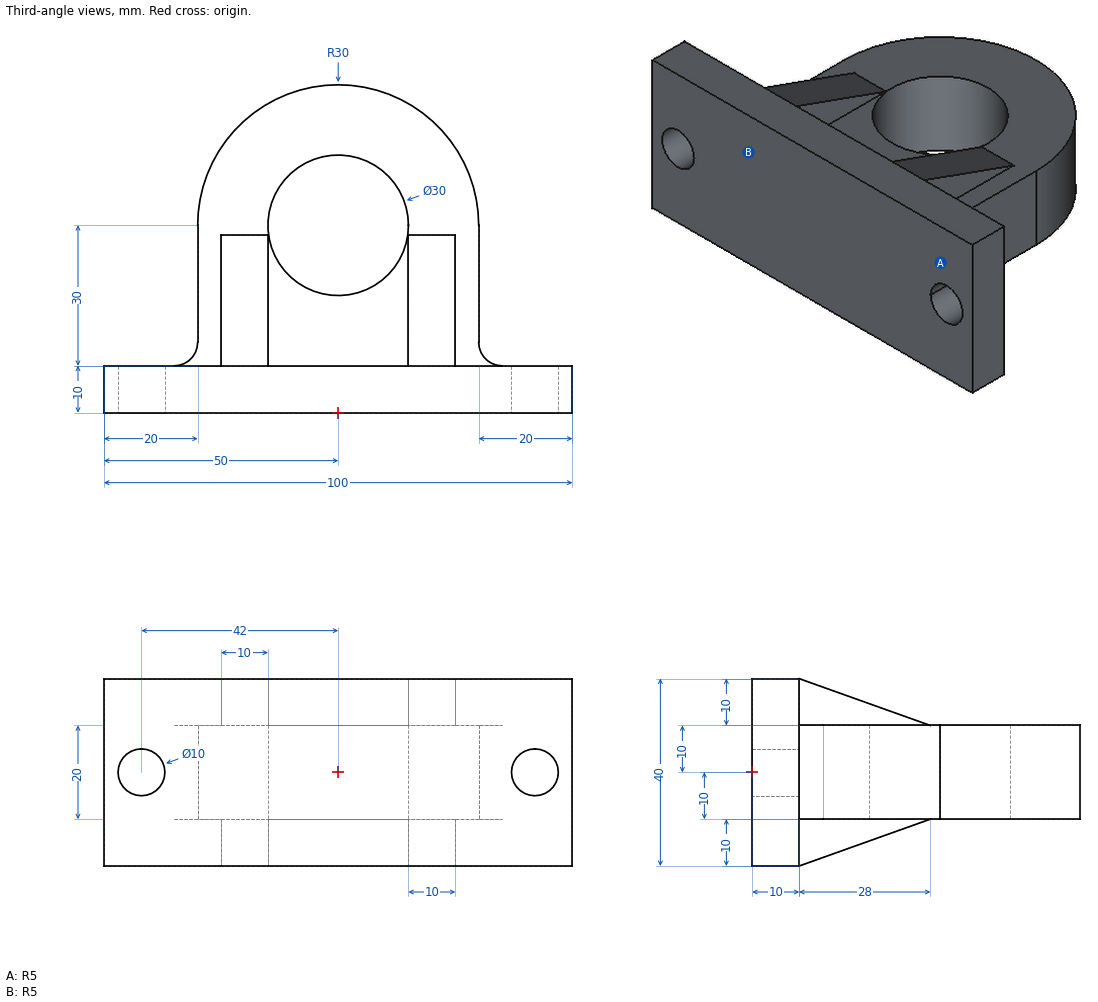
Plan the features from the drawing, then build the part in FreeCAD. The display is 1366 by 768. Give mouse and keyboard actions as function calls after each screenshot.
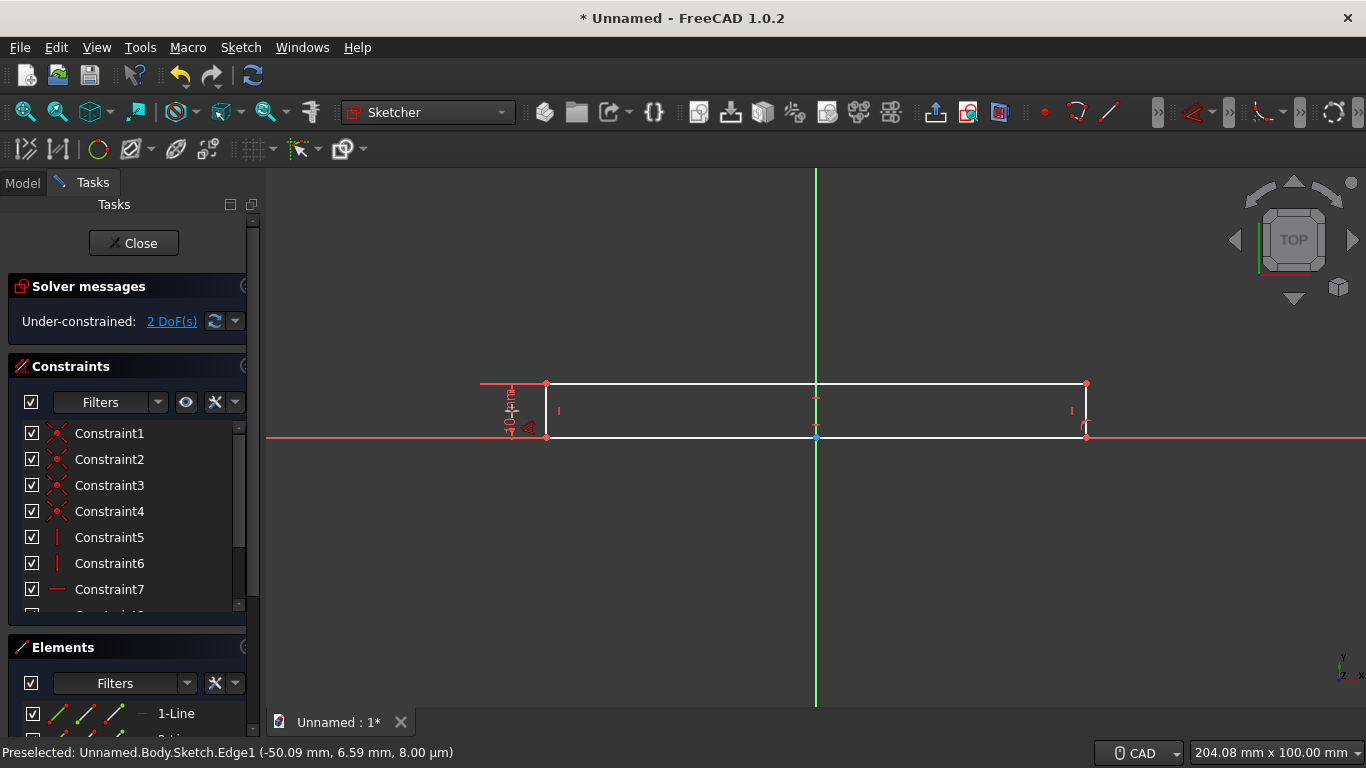
click(708, 438)
click(692, 472)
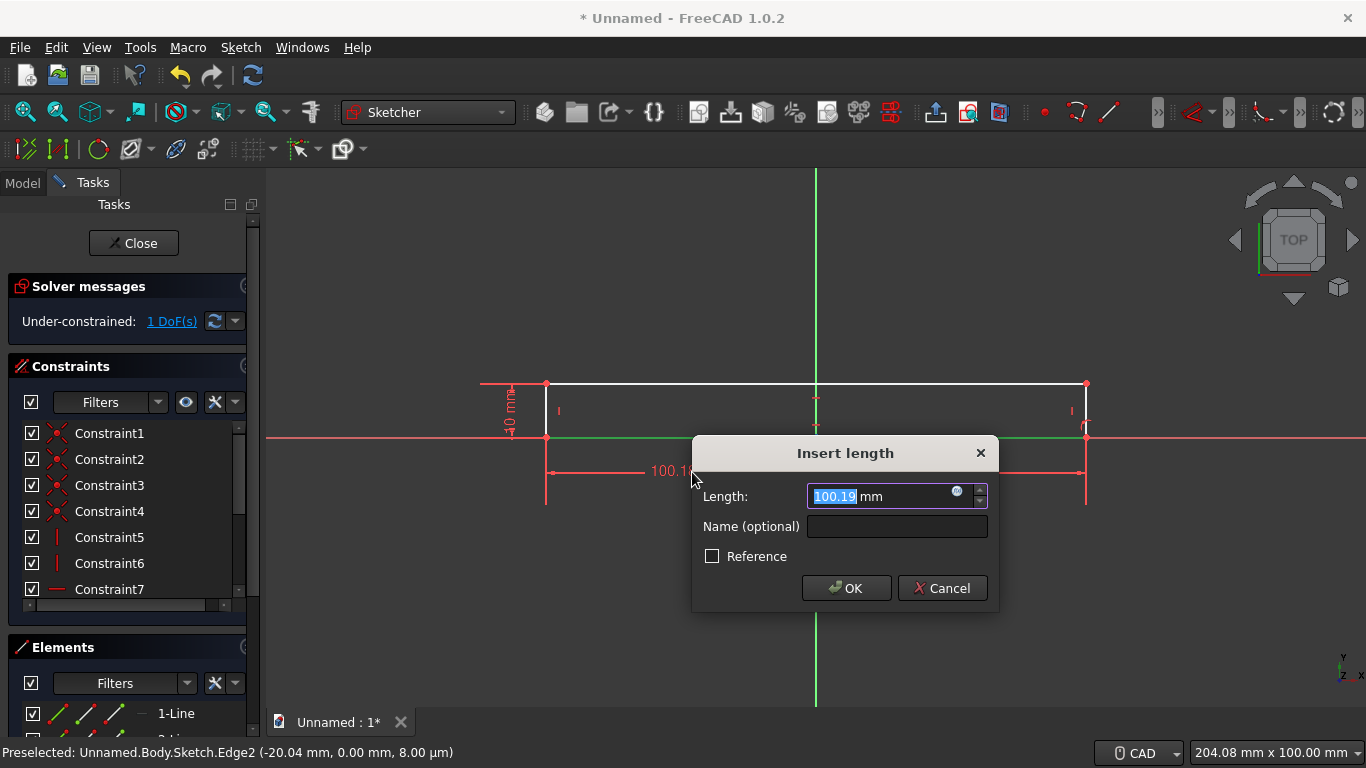
text(100)
key(Return)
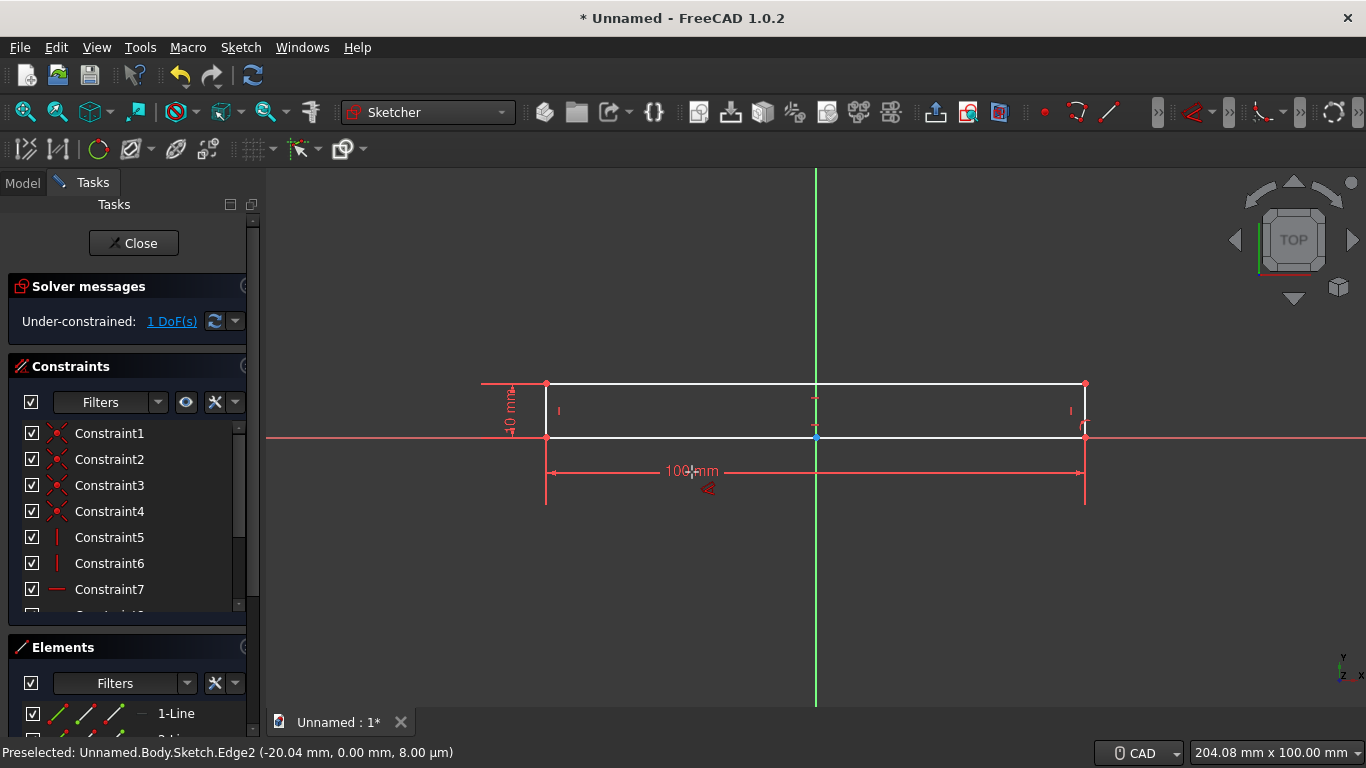
click(546, 384)
click(619, 472)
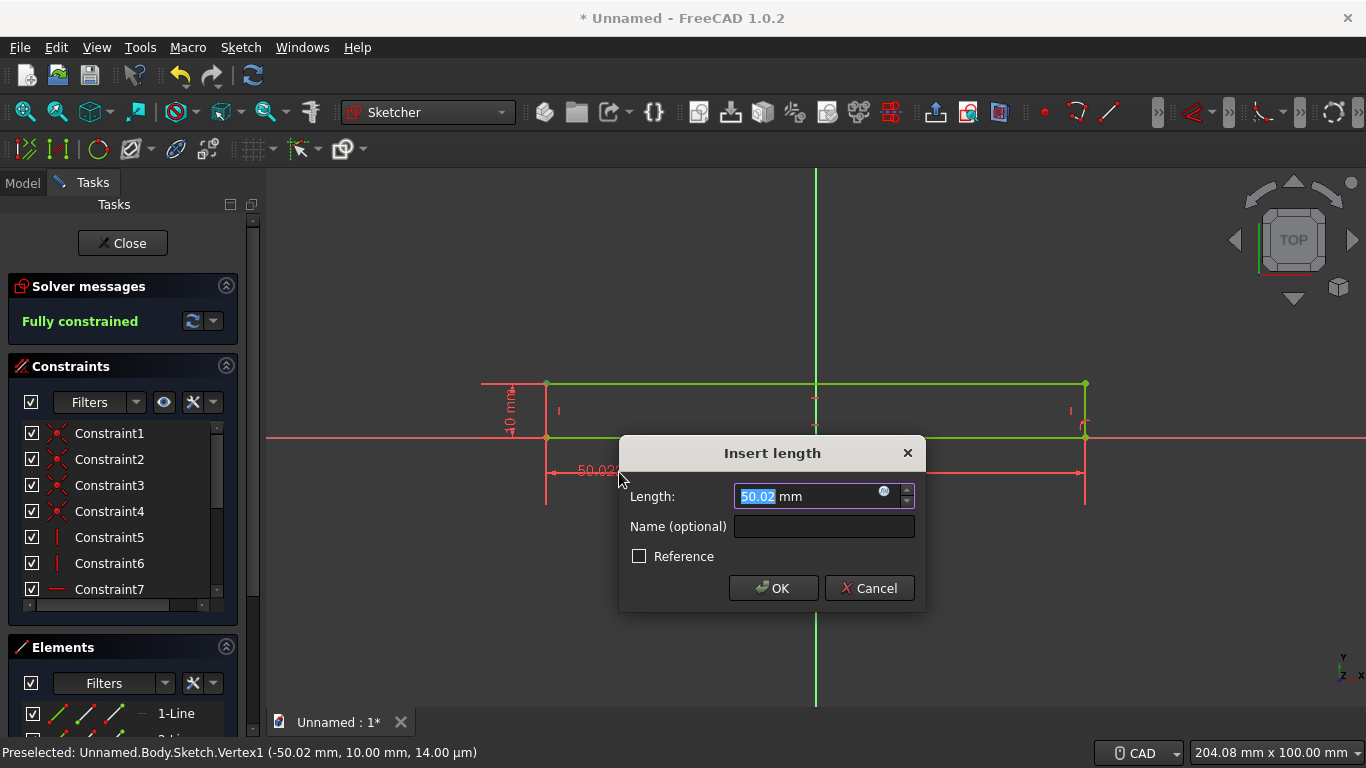
text(50)
key(Return)
key(Escape)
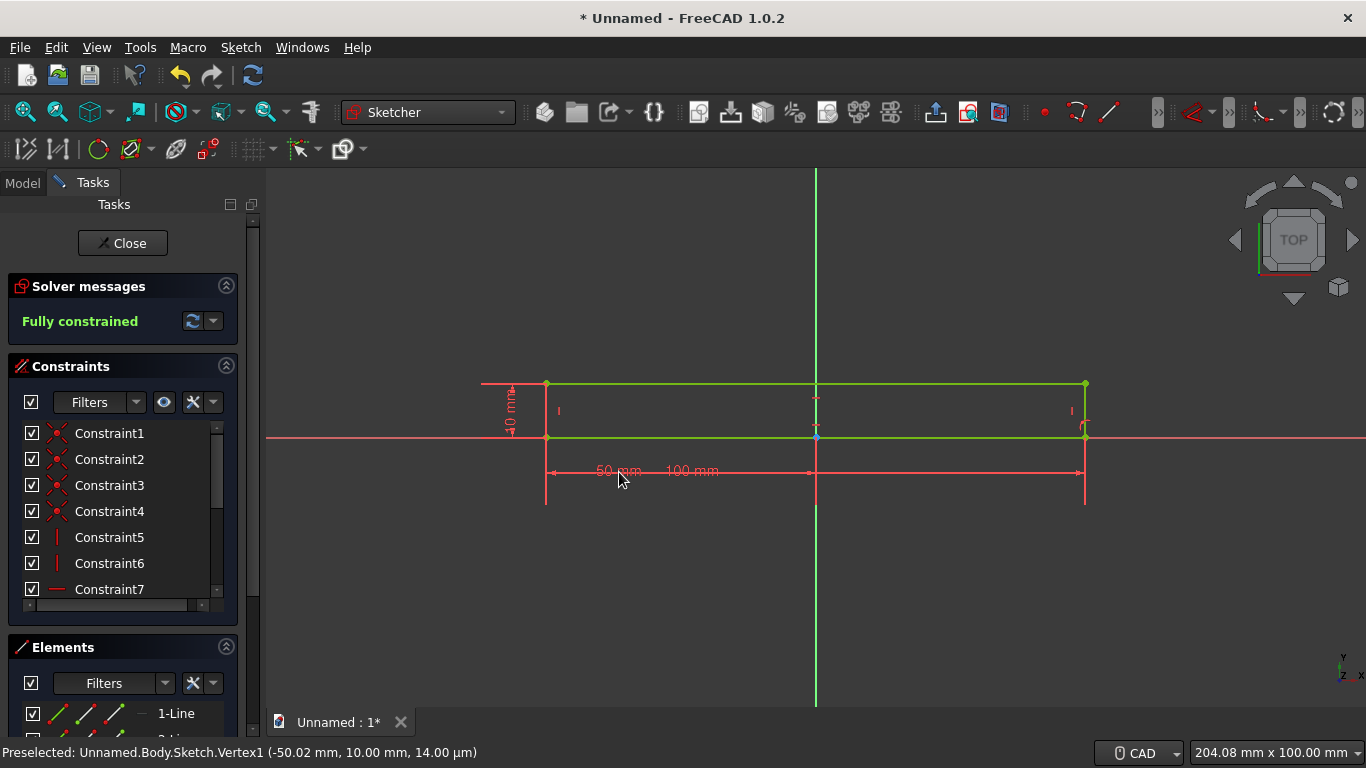
click(123, 243)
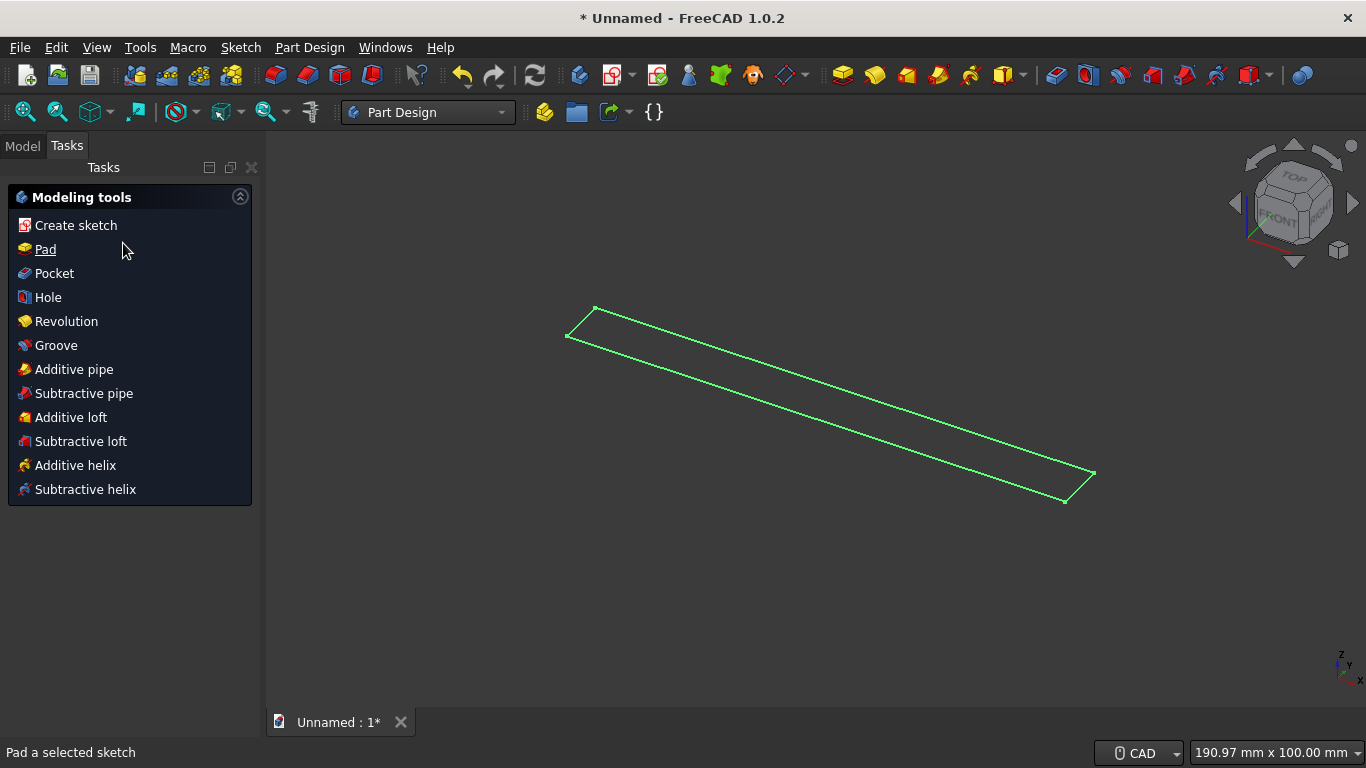
click(844, 76)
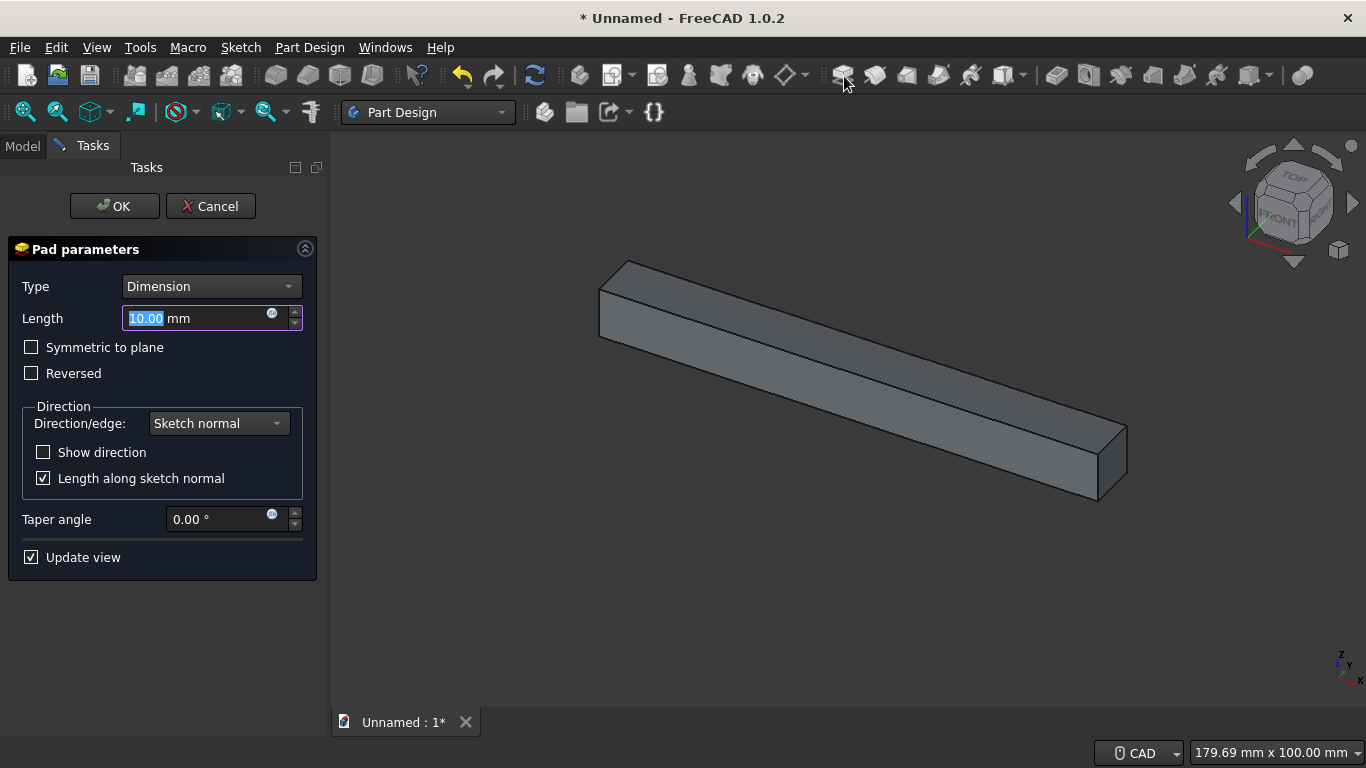
text(40)
key(Tab)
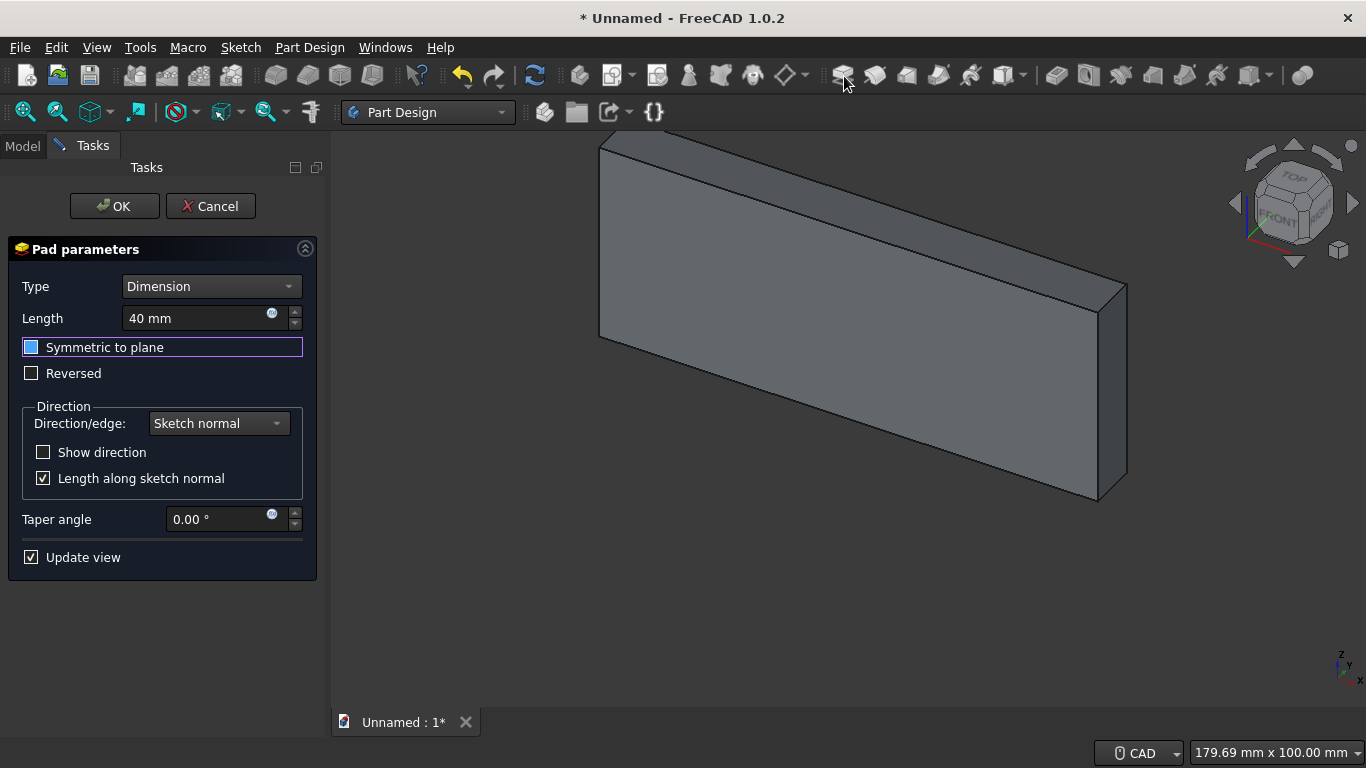
click(30, 347)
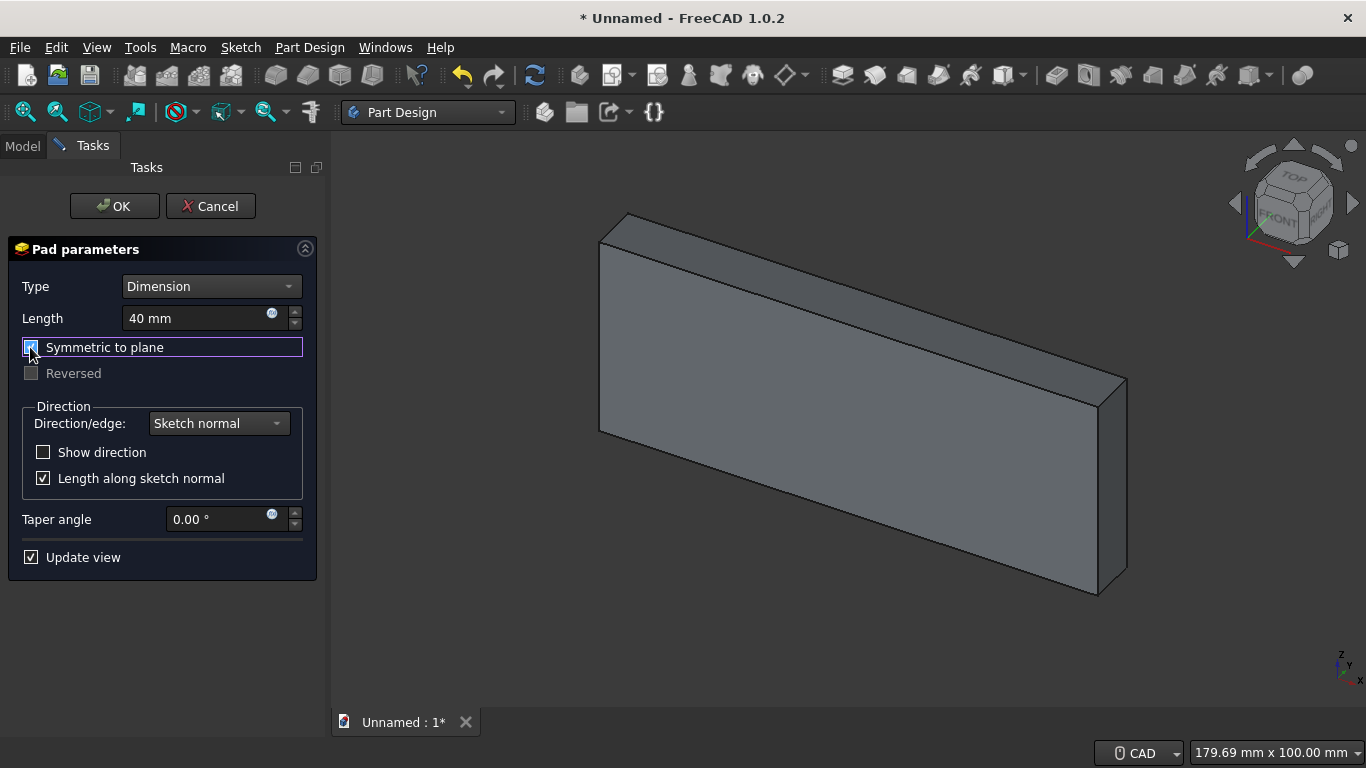
click(115, 206)